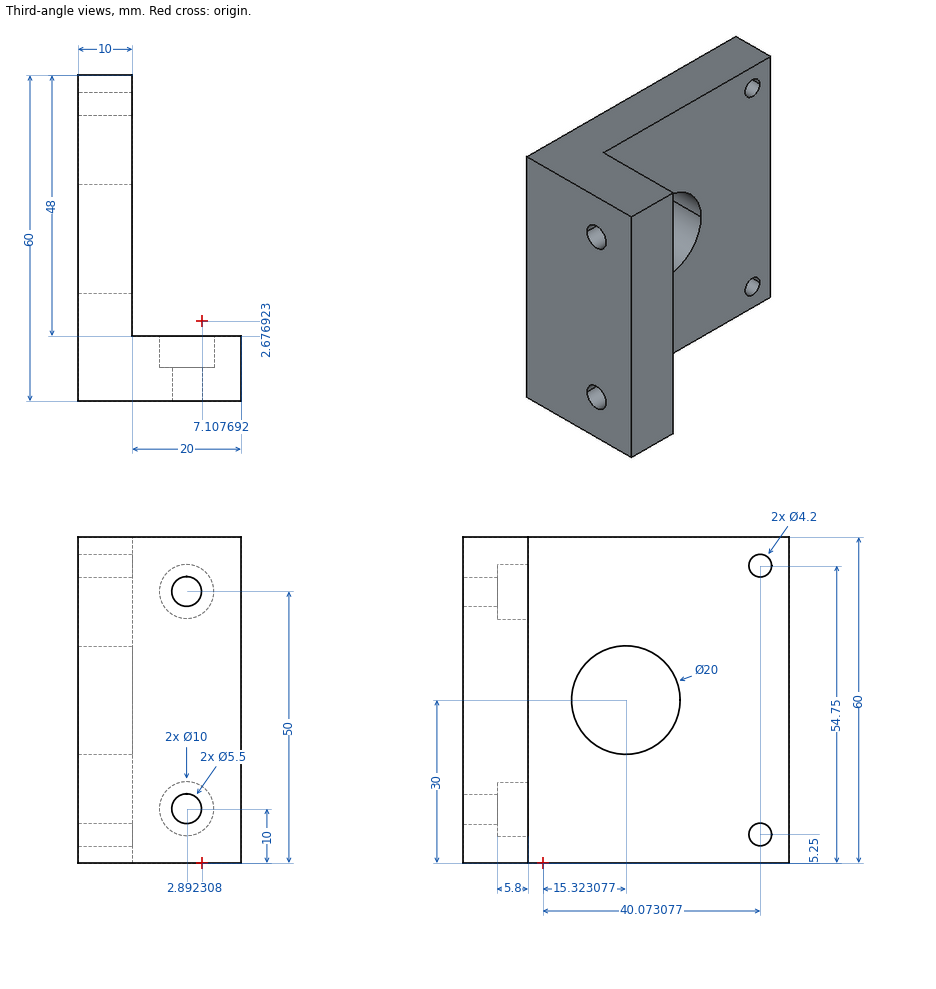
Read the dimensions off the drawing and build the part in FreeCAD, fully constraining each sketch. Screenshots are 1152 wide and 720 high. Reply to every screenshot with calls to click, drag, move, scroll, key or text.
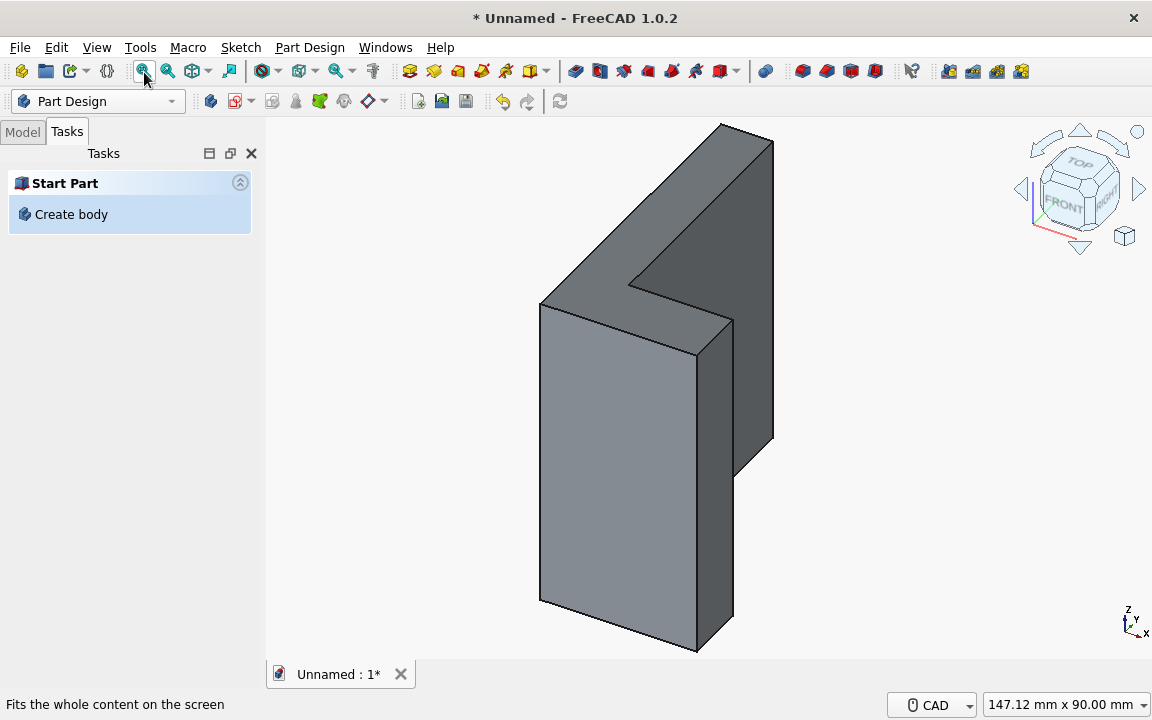
click(722, 298)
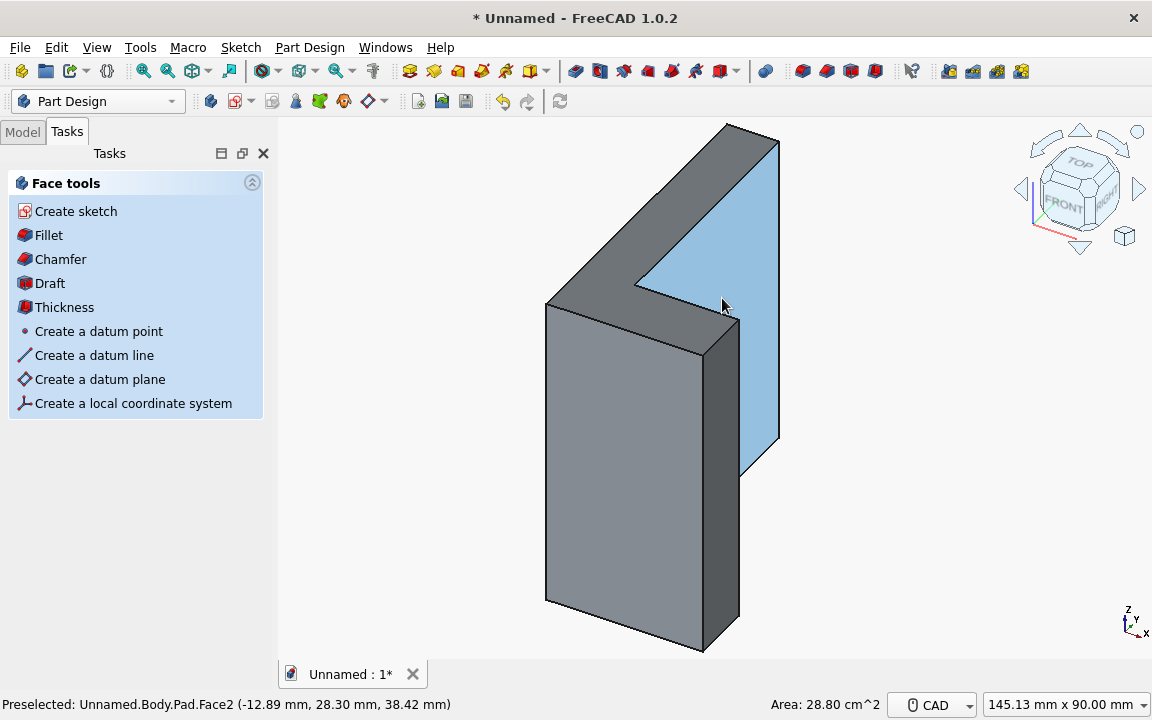
click(236, 102)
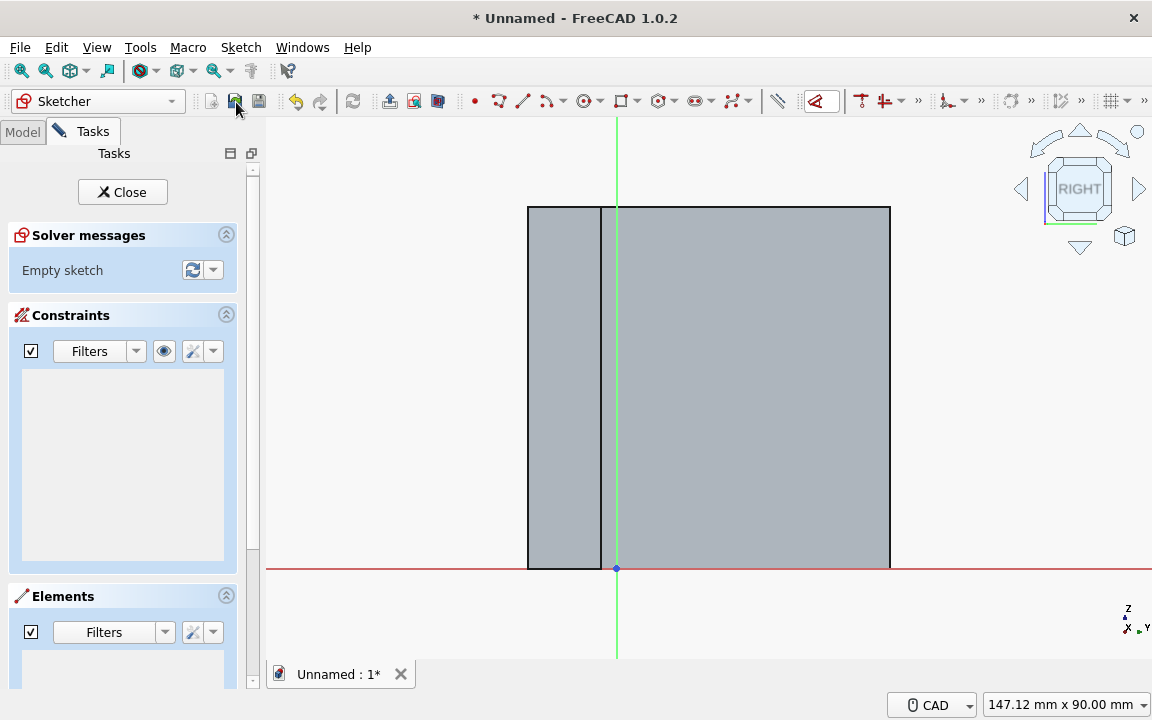
scroll(800, 571, up, 2)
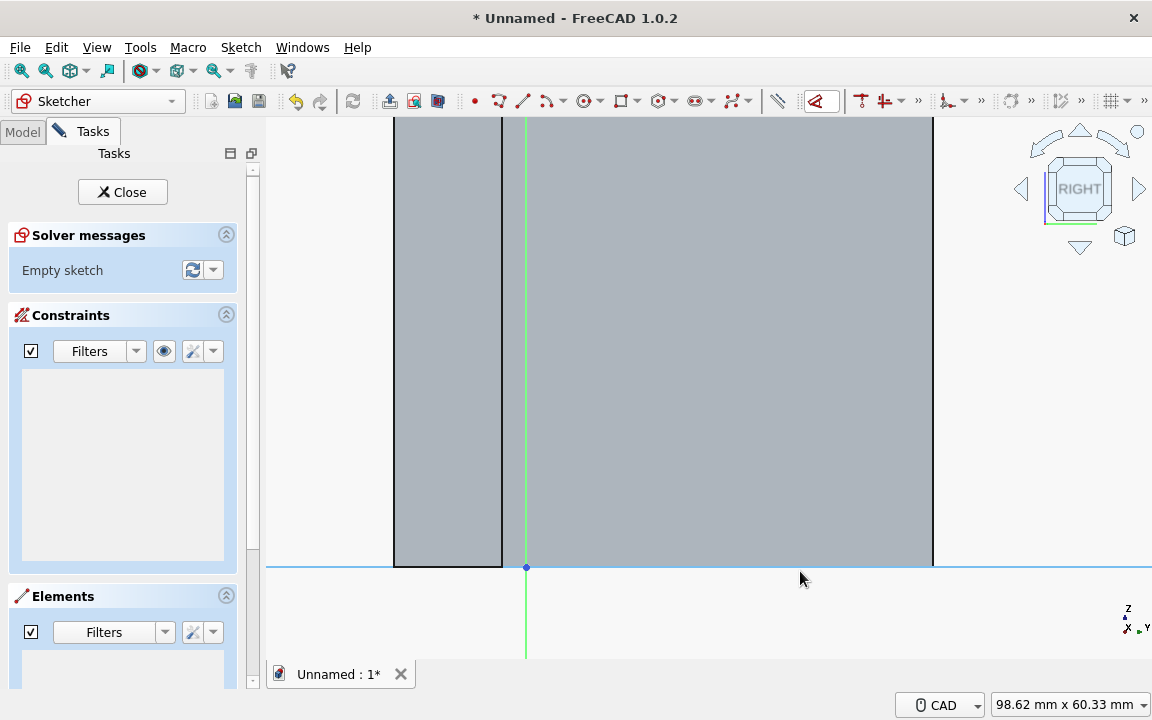
click(584, 102)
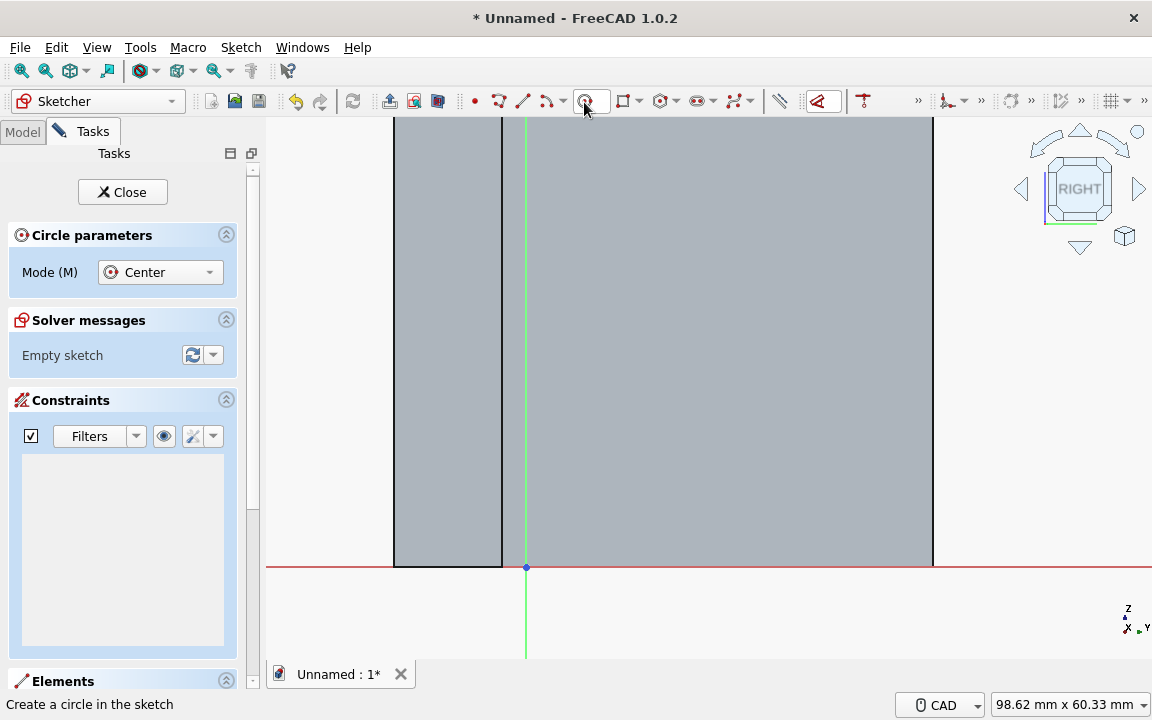
click(664, 298)
move(727, 234)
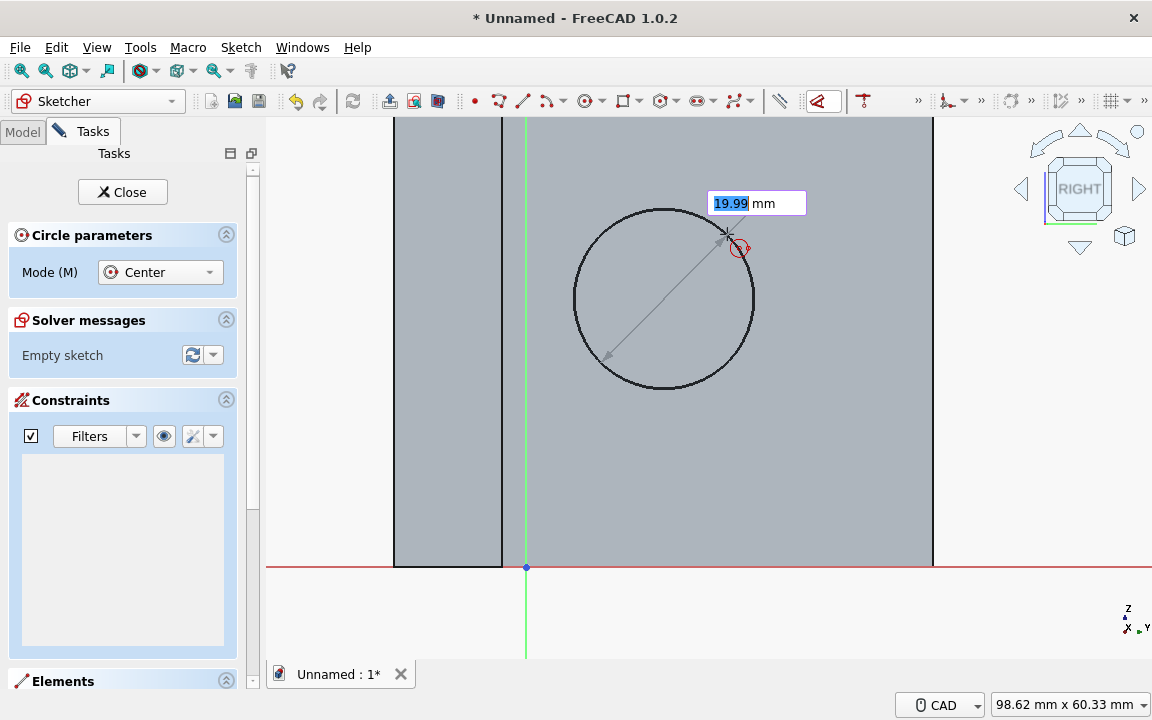
text(20)
key(Return)
key(Escape)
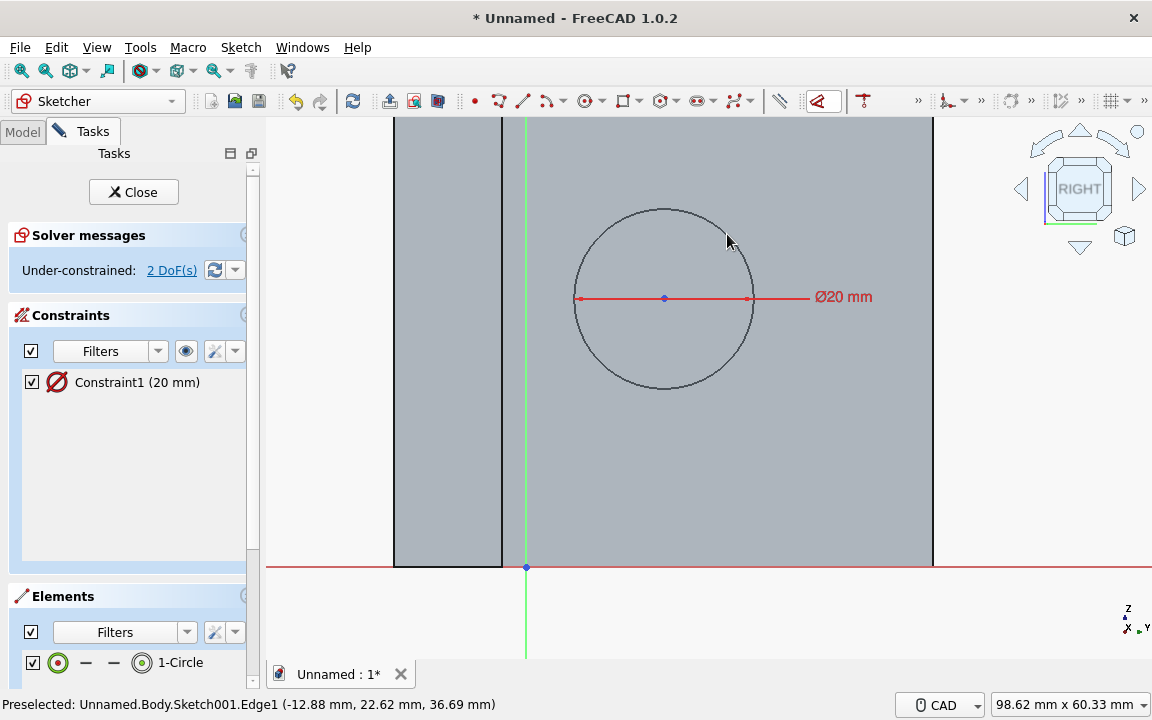
click(664, 299)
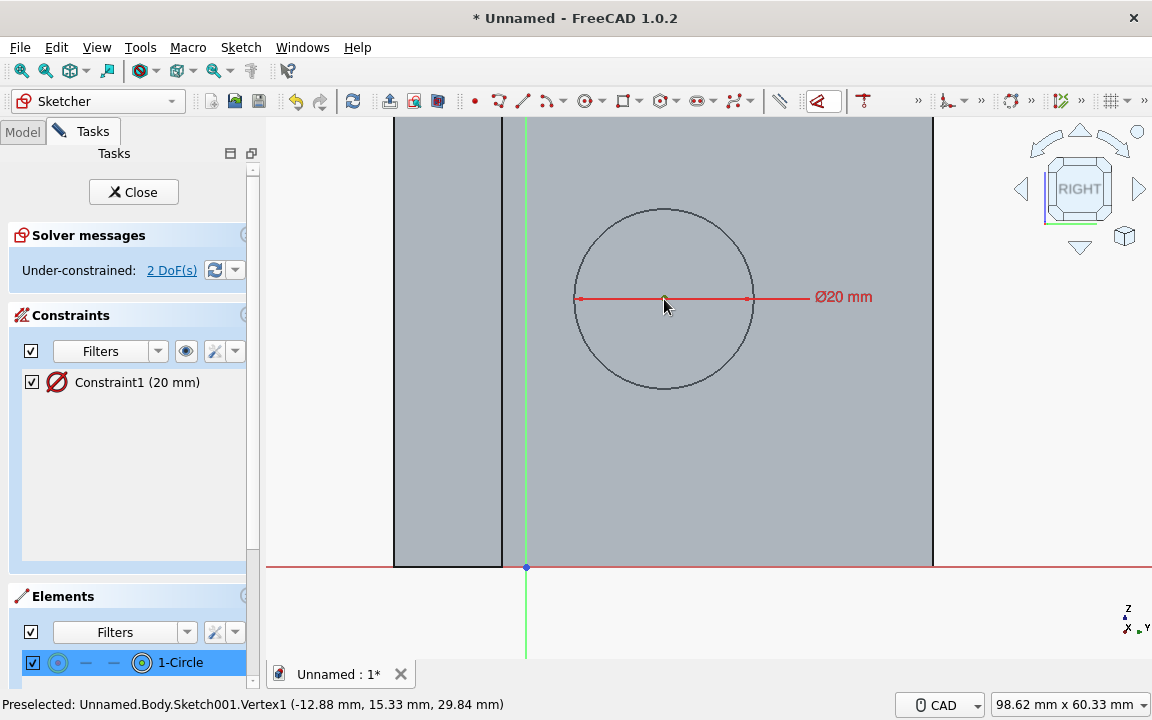
click(836, 102)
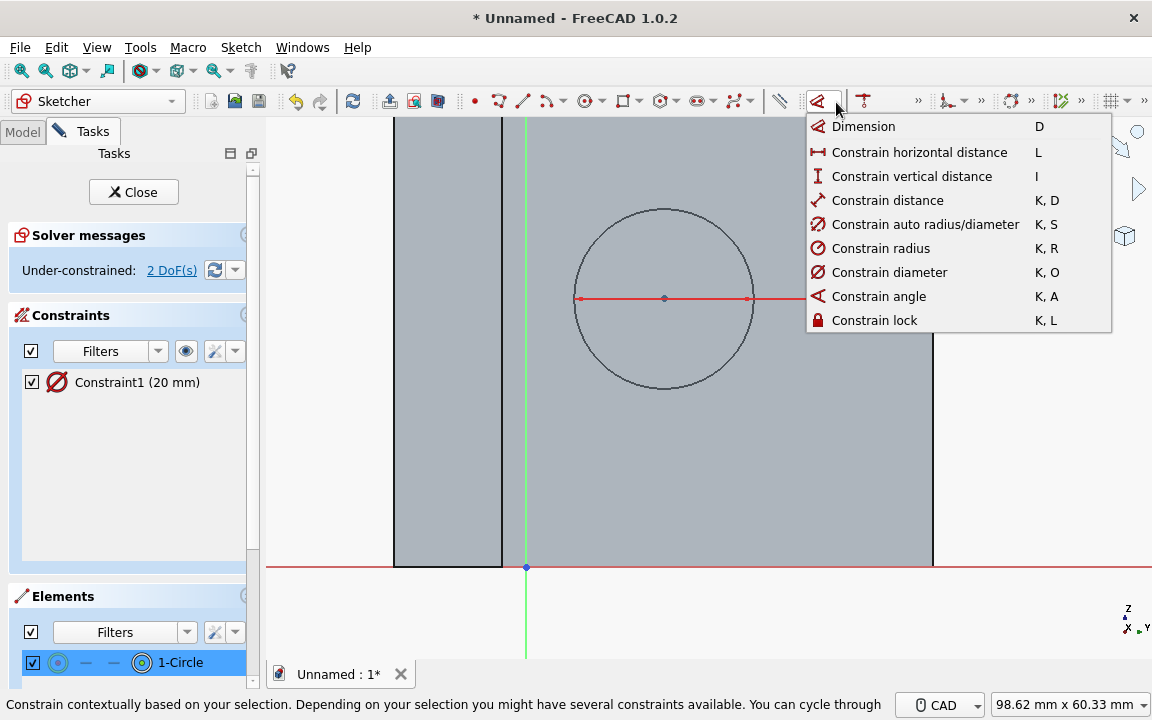
click(959, 176)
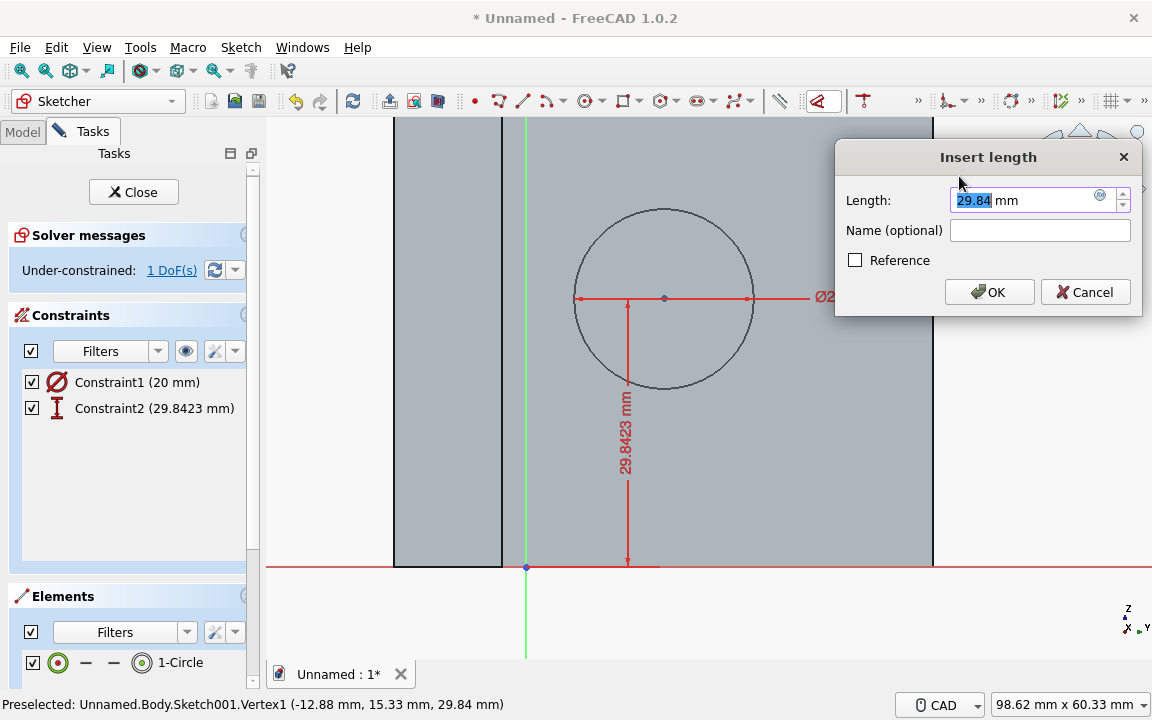
text(30)
key(Return)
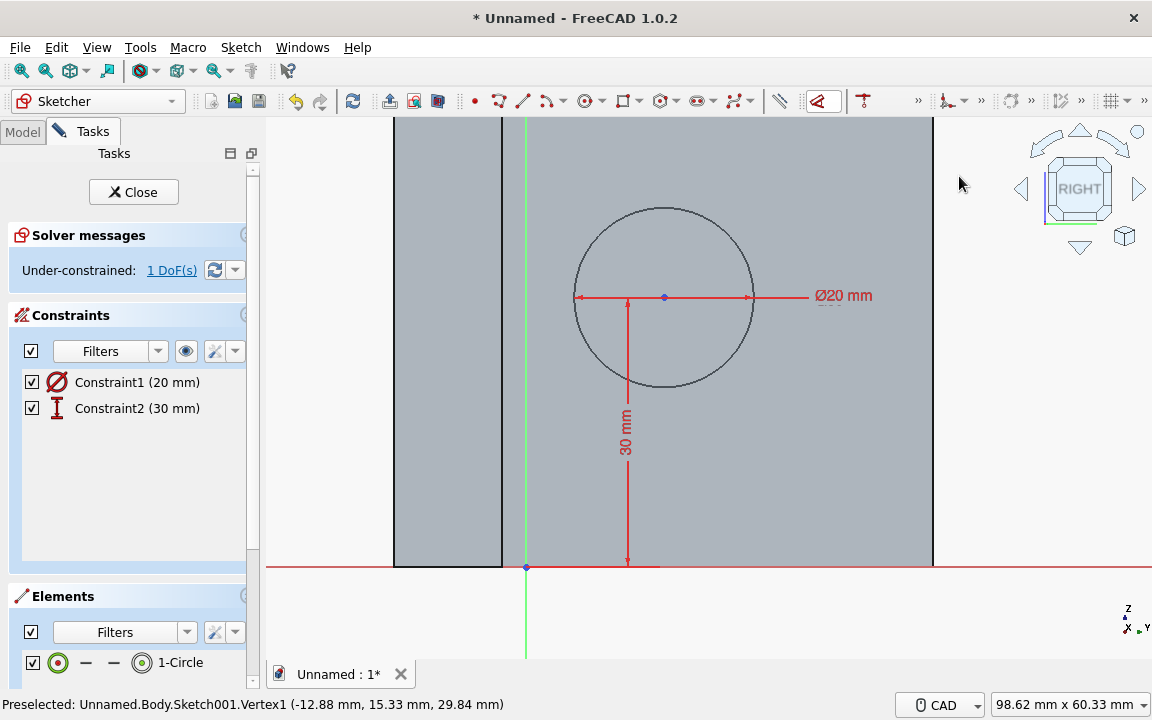
click(664, 298)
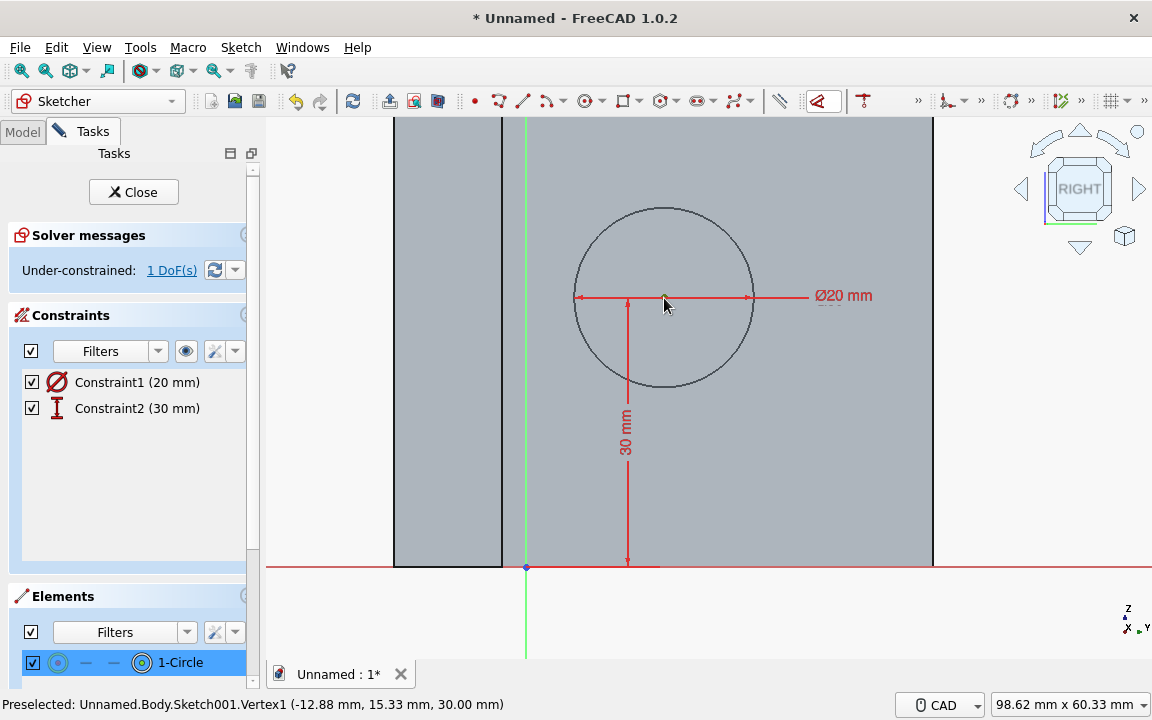
click(836, 102)